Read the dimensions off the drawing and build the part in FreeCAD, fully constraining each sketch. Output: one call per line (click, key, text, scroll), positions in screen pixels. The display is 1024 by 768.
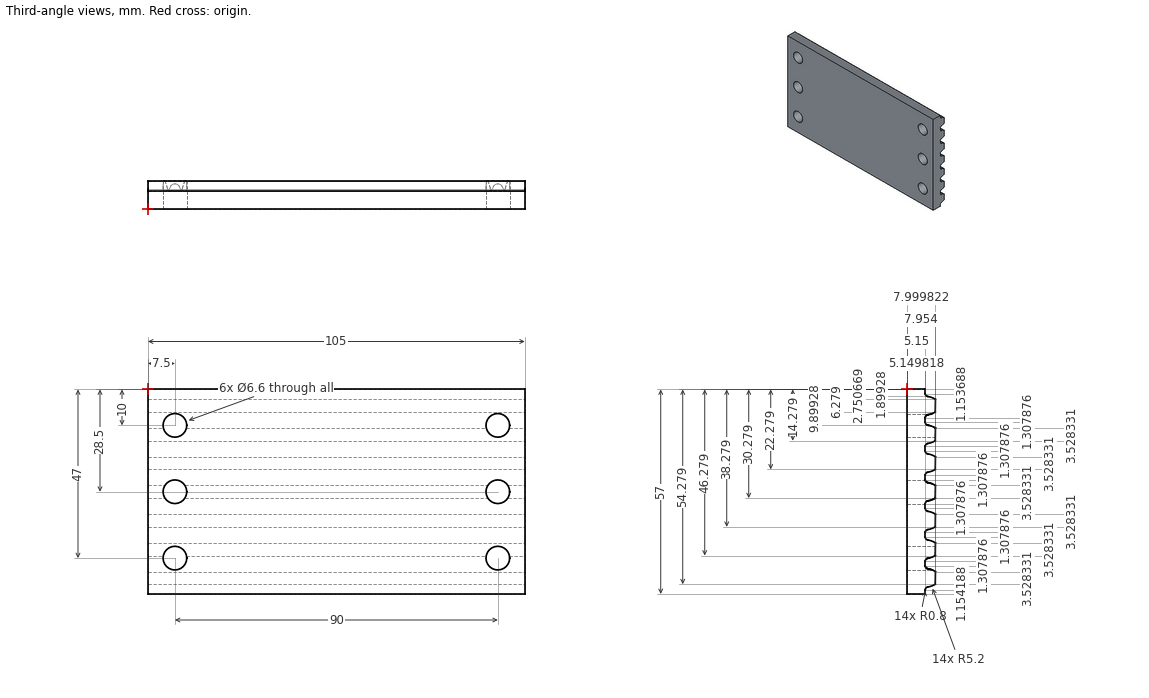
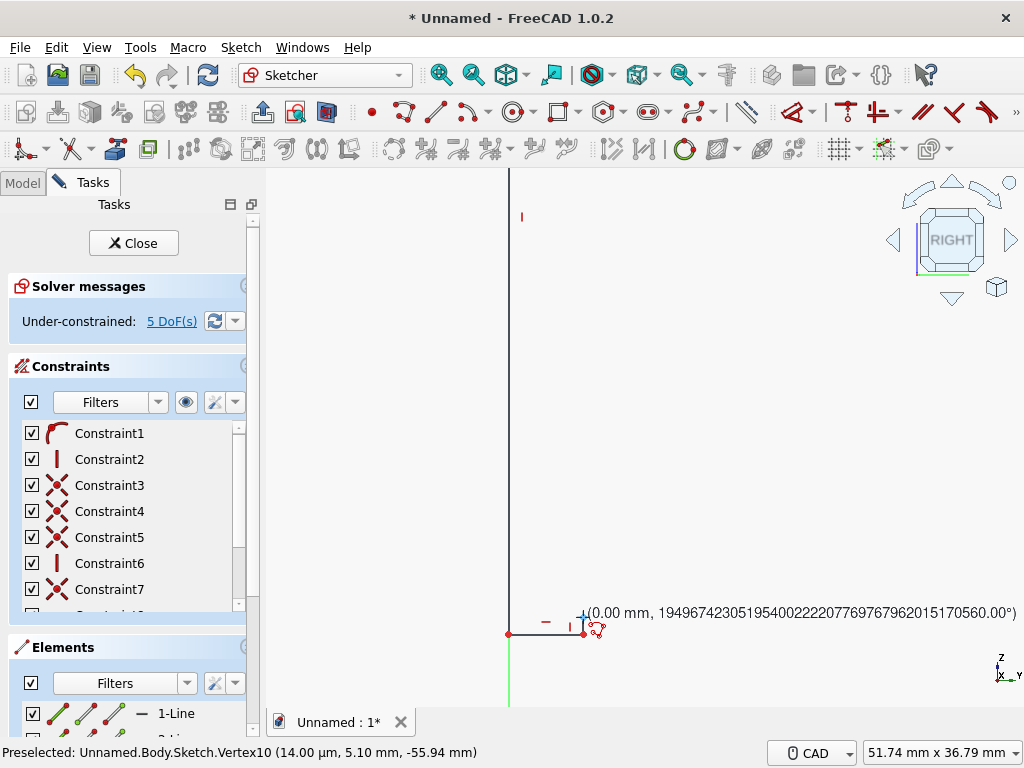
click(436, 112)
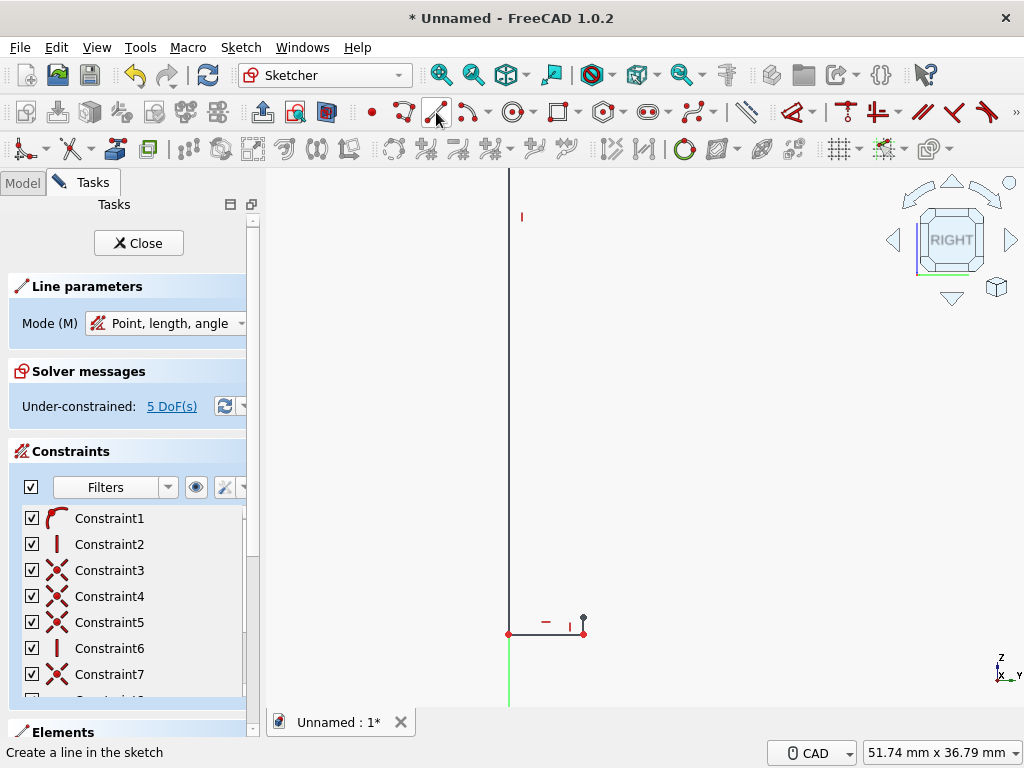
click(625, 594)
click(629, 542)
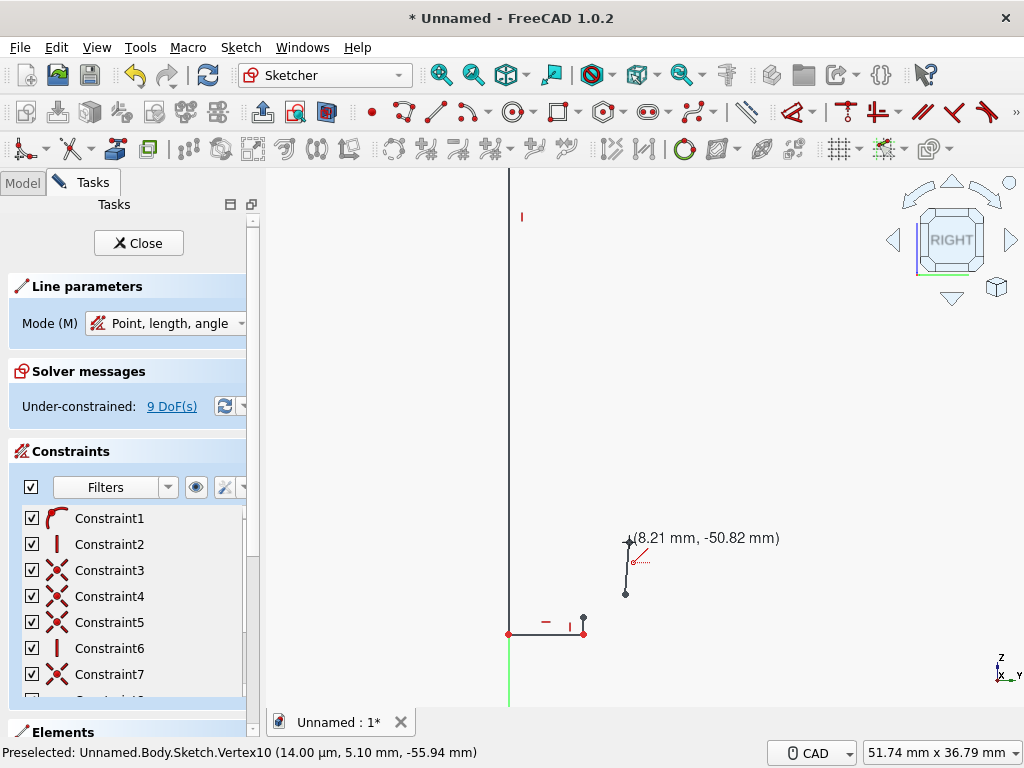
click(584, 519)
click(584, 499)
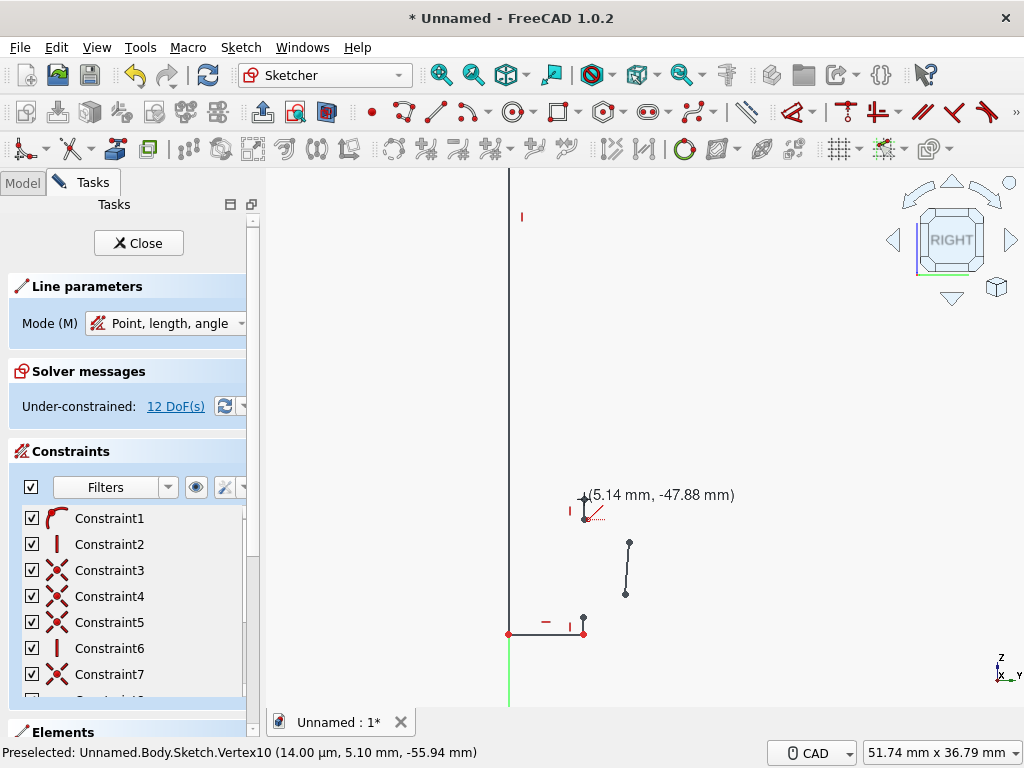
click(625, 476)
click(629, 425)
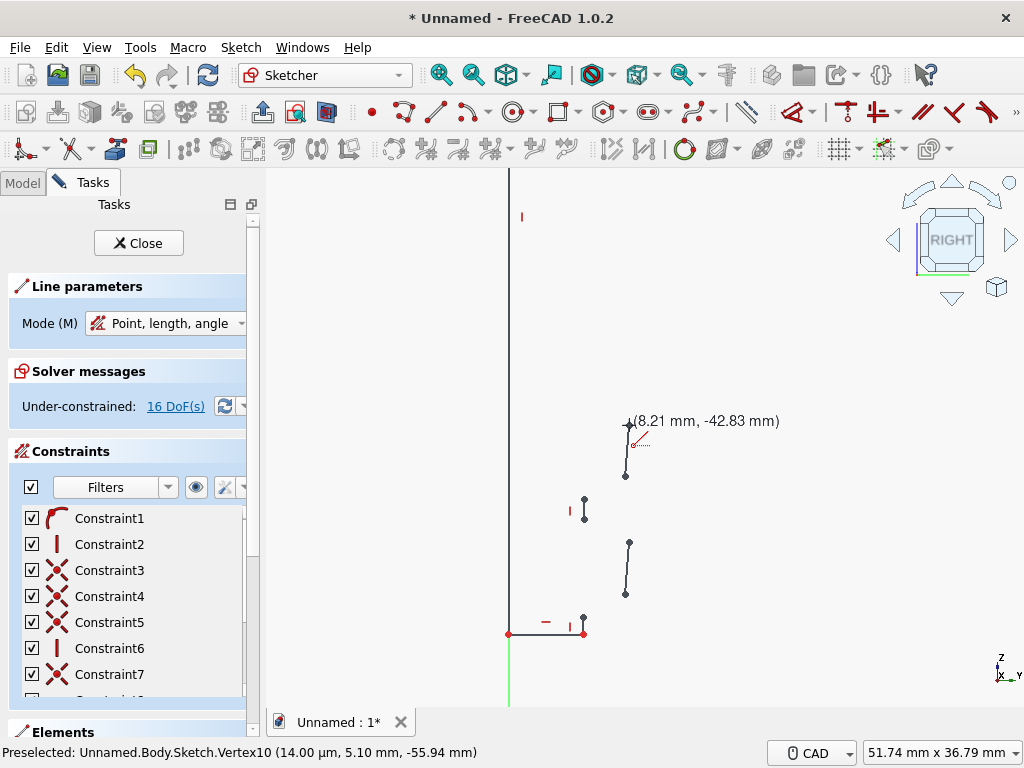
click(584, 401)
click(584, 382)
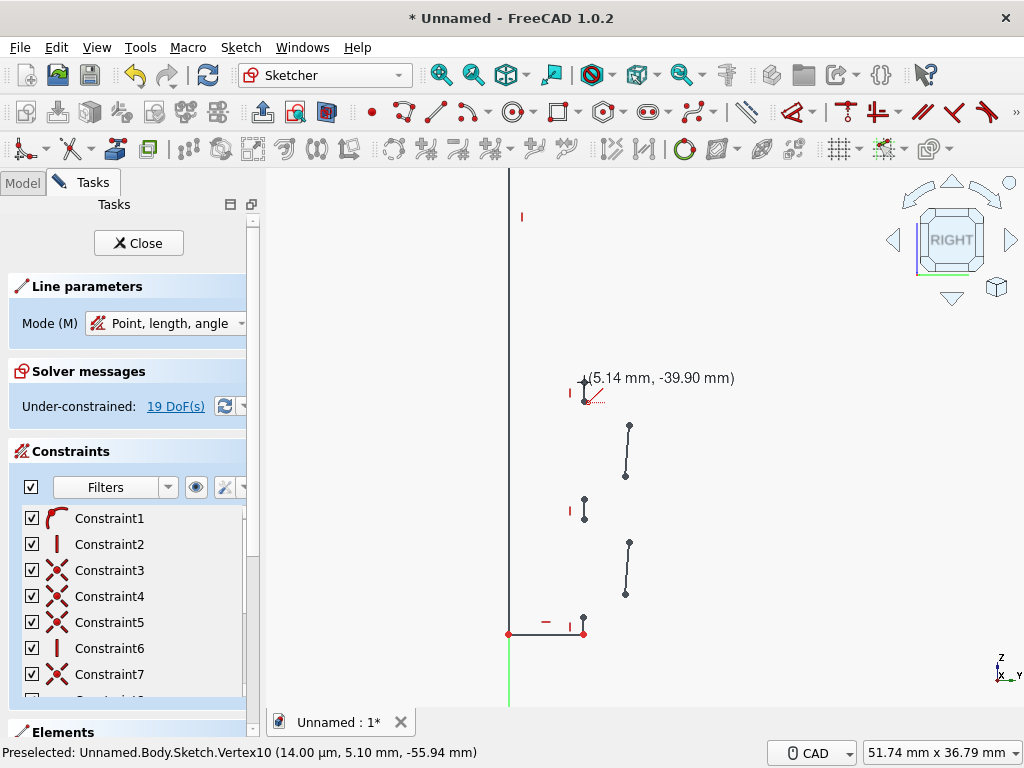
click(625, 359)
click(629, 308)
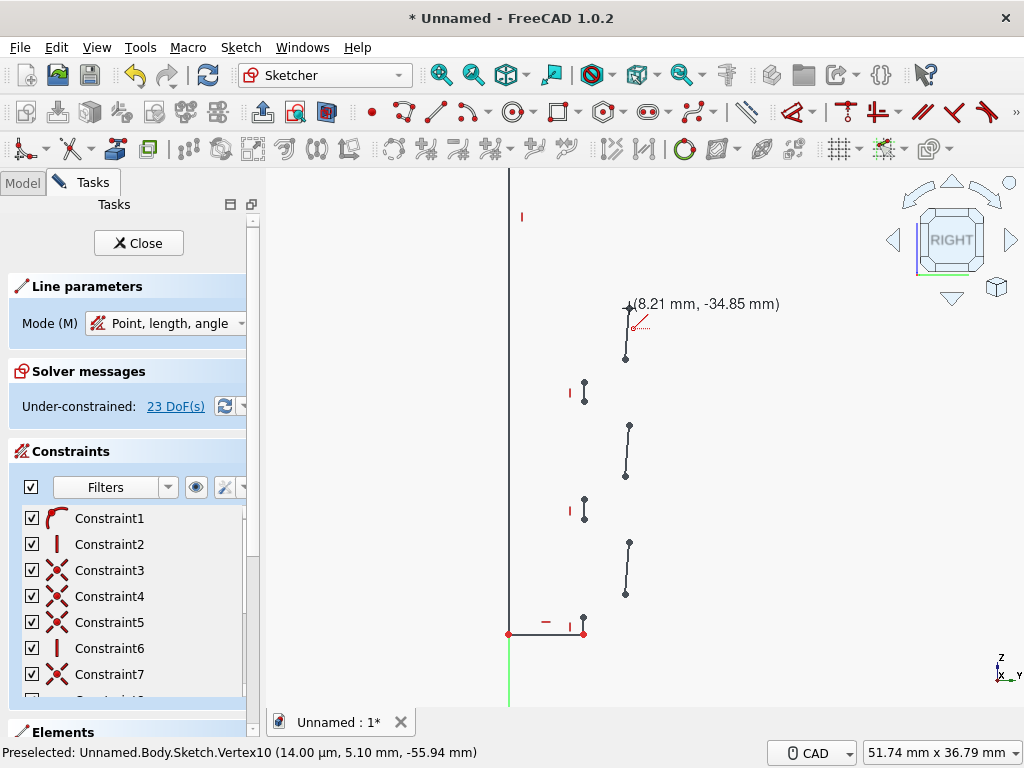
click(584, 284)
click(584, 265)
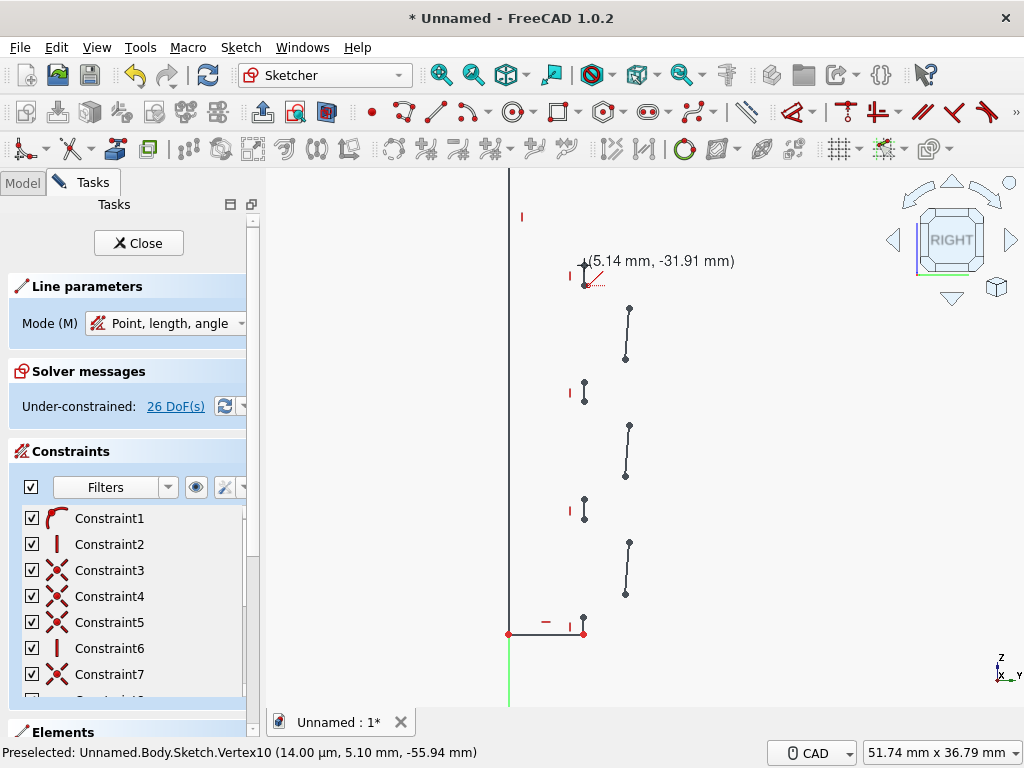
click(625, 242)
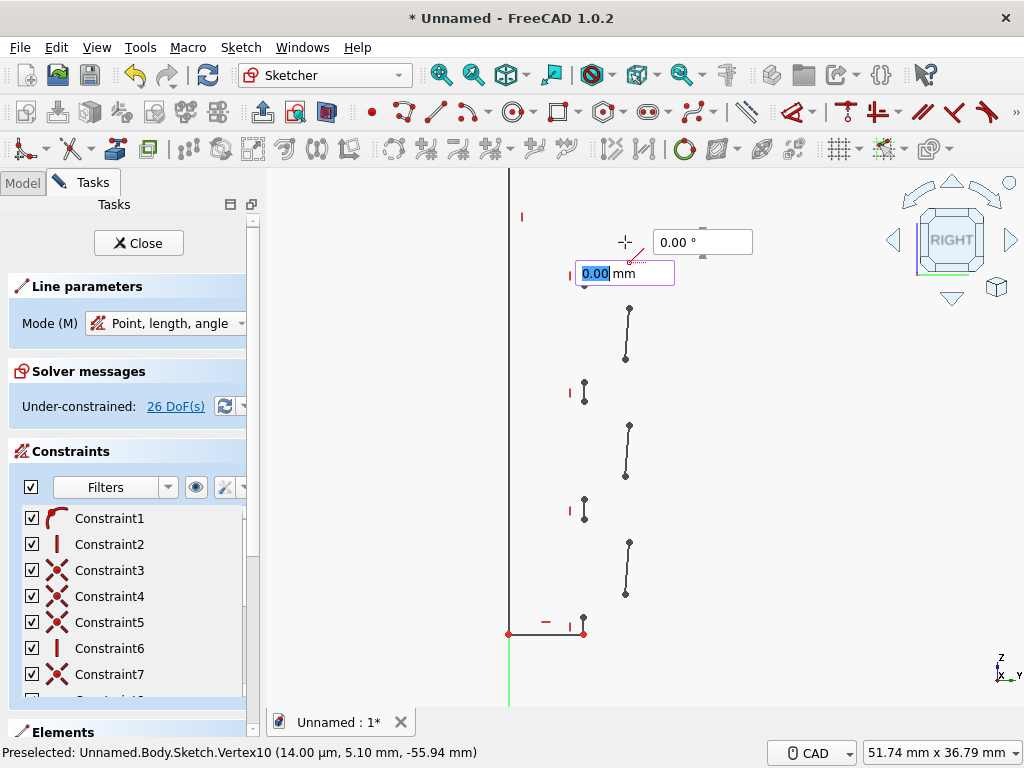
scroll(584, 618, down, 4)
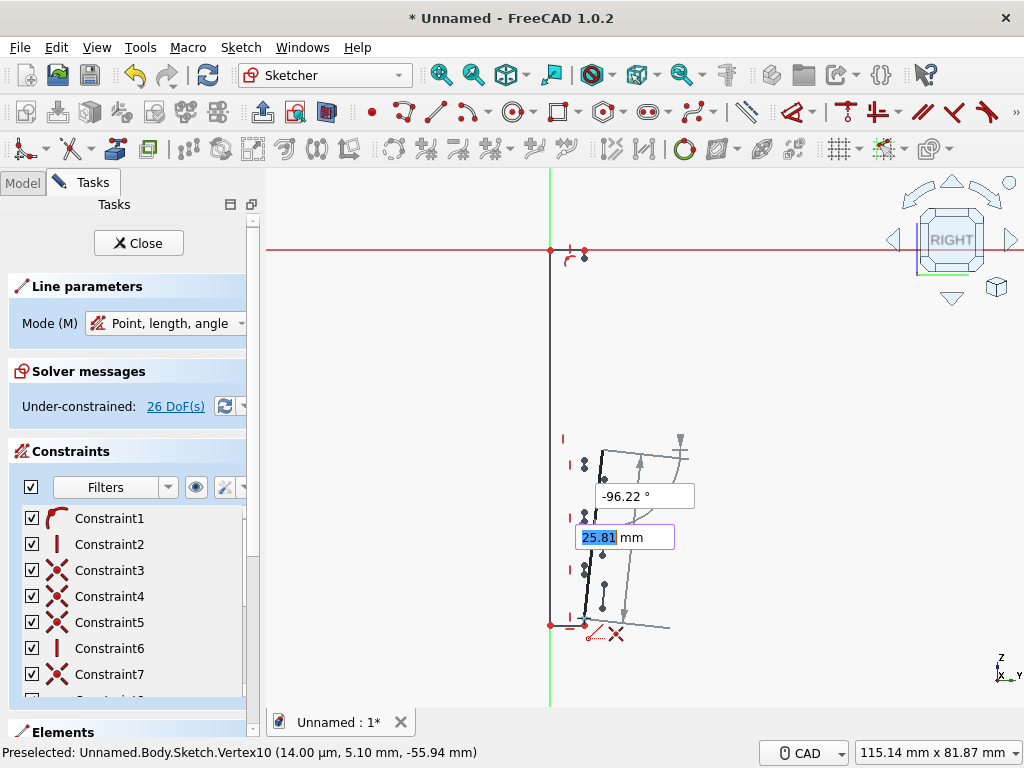
click(605, 426)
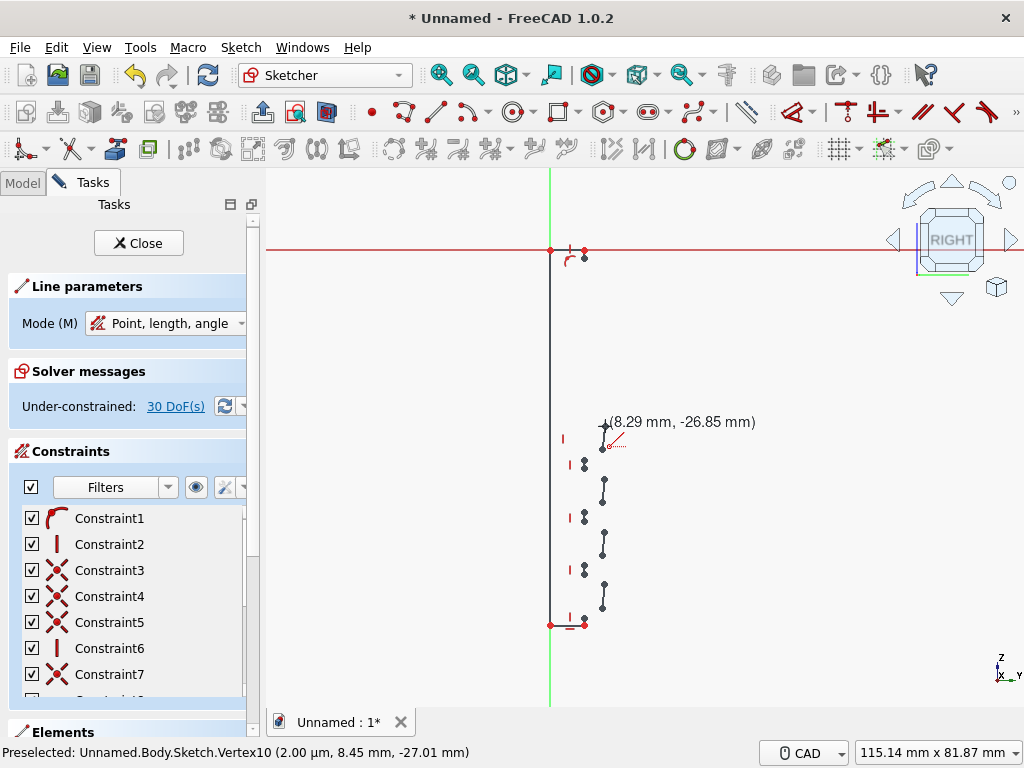
click(584, 416)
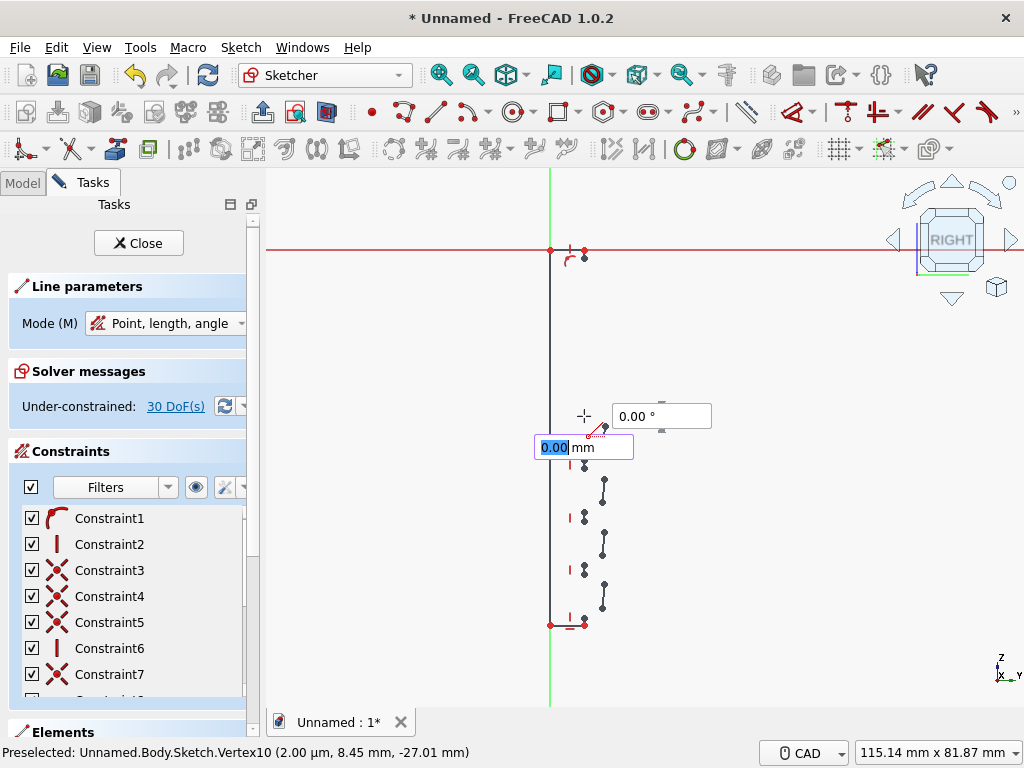
scroll(584, 407, up, 4)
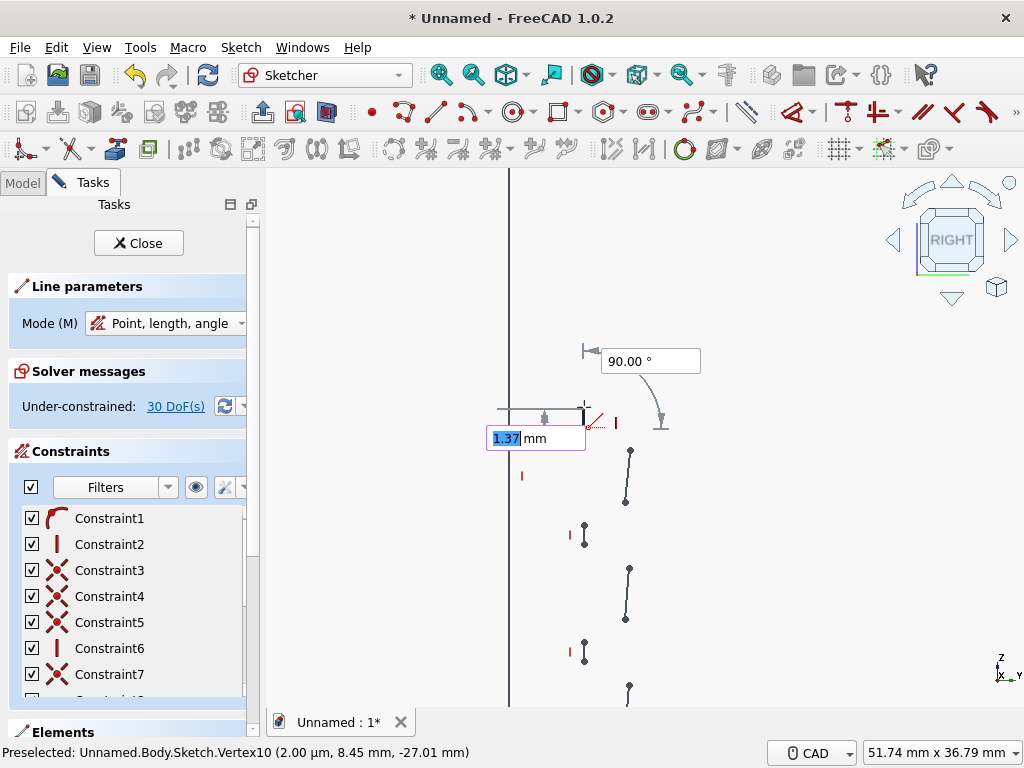
click(583, 407)